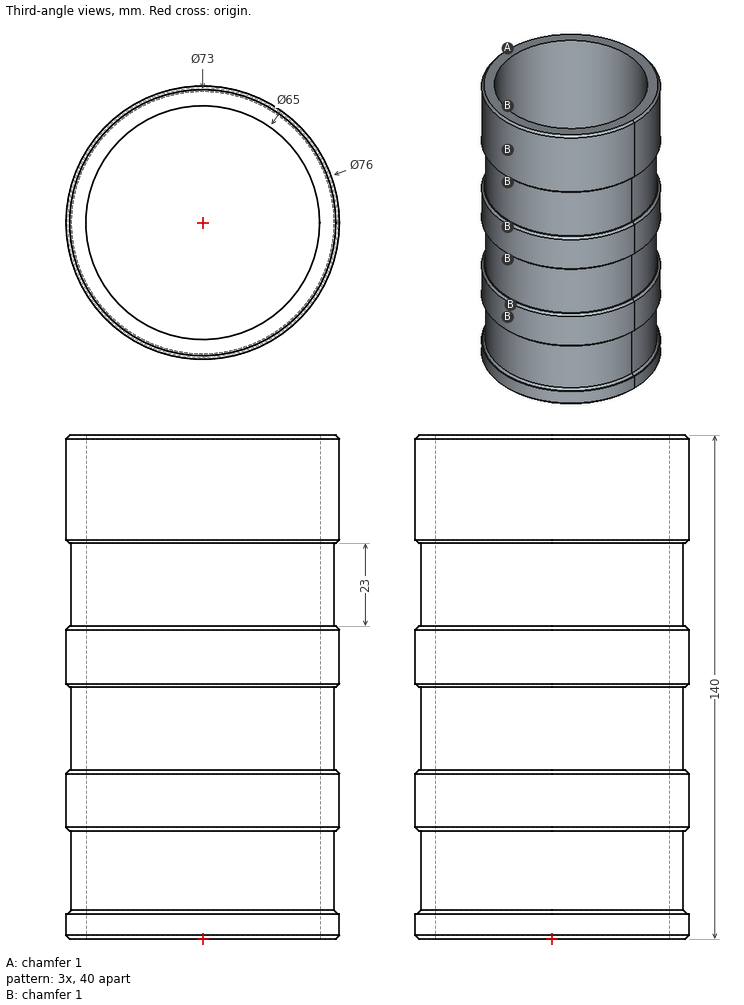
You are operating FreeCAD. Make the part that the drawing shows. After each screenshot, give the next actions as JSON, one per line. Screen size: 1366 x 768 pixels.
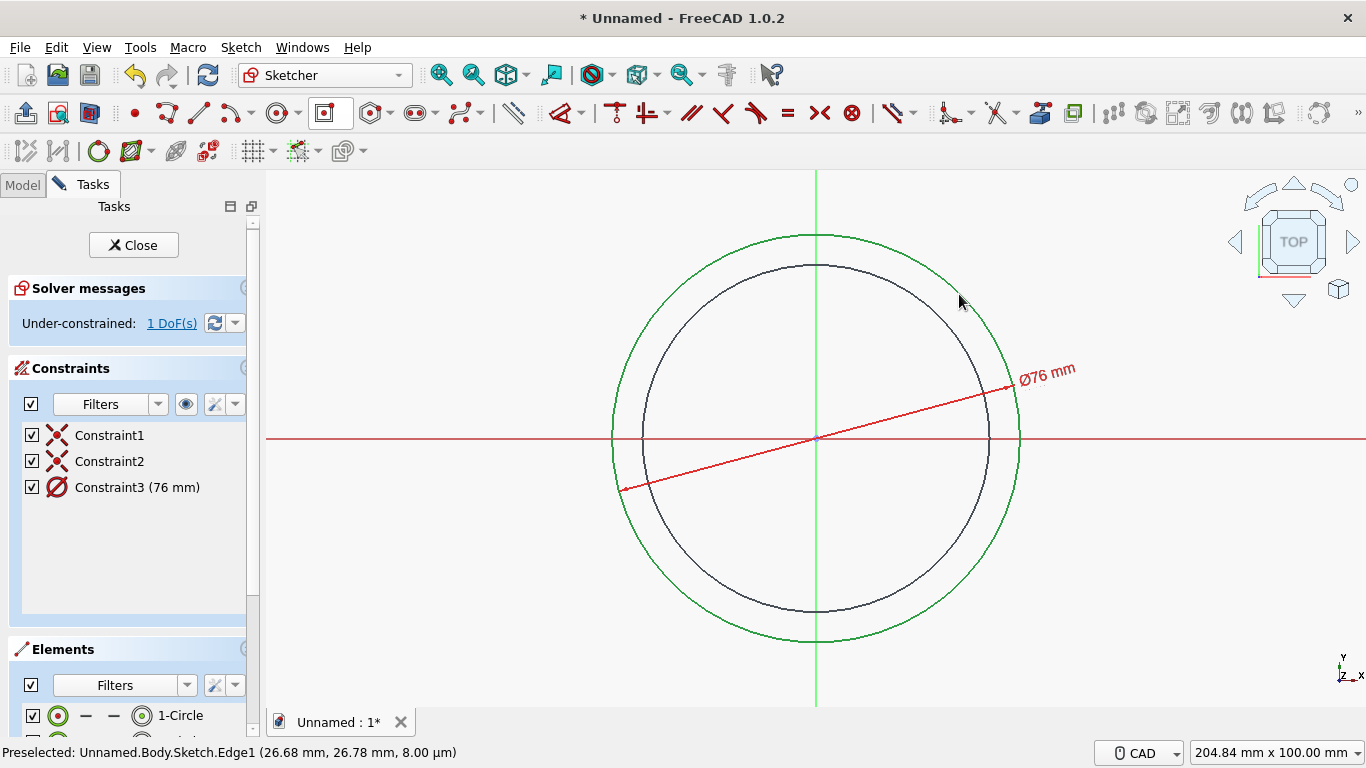
{"action": "left_click", "coordinate": [938, 315]}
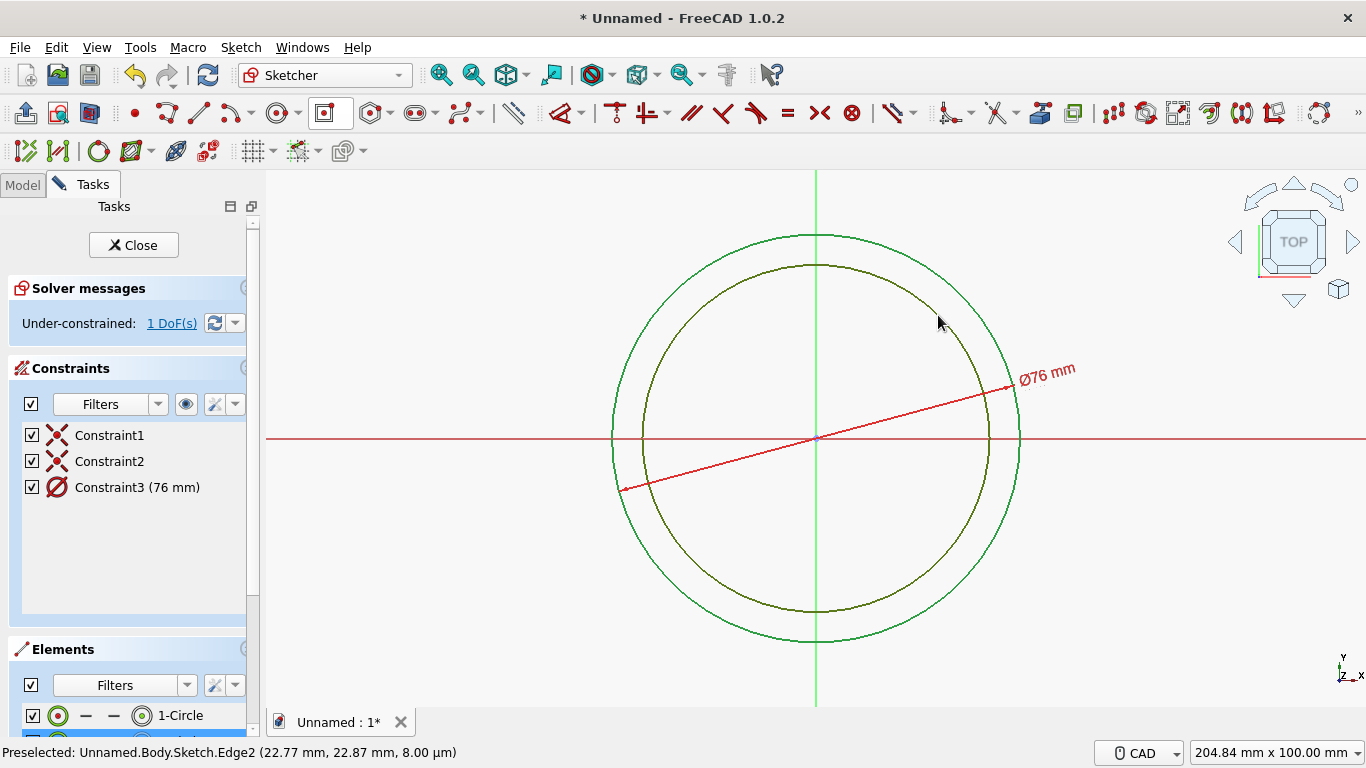
{"action": "key", "text": "k o"}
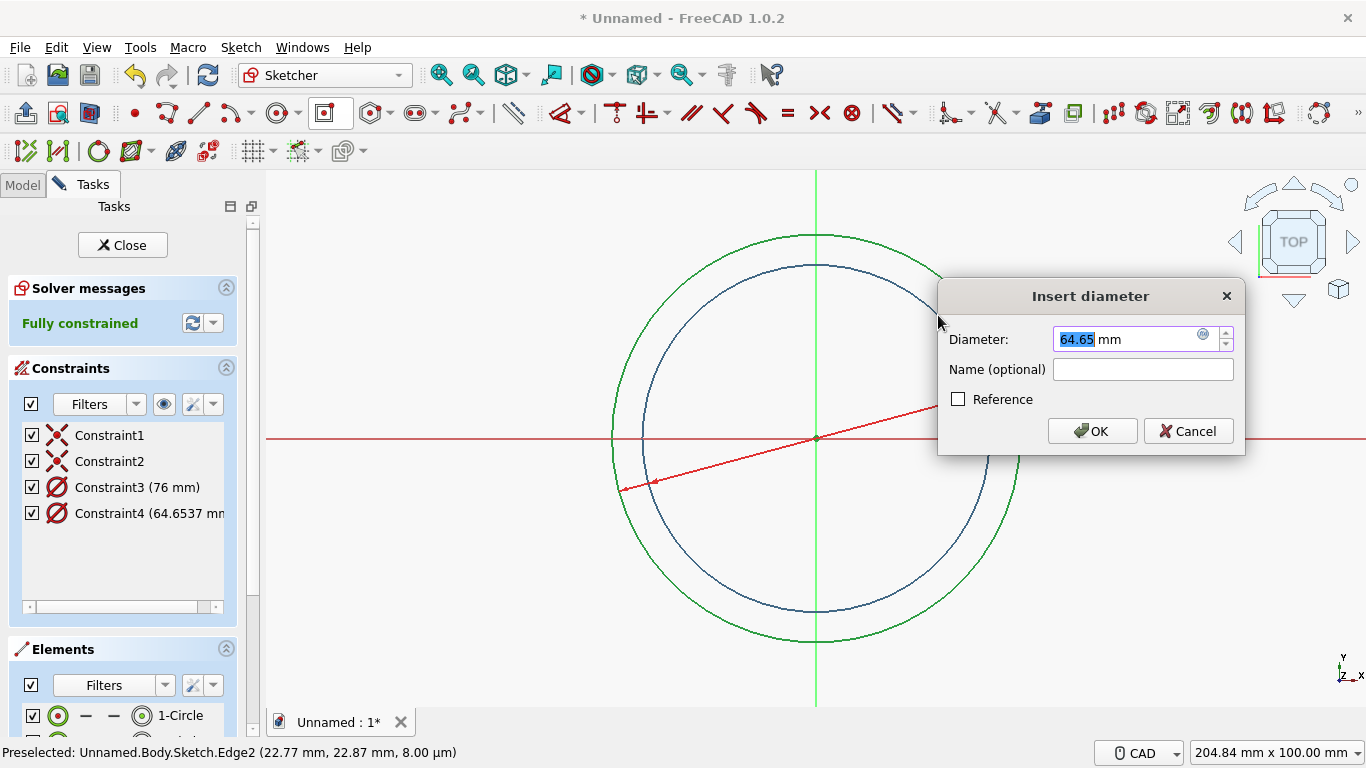
{"action": "type", "text": "65"}
{"action": "key", "text": "Return"}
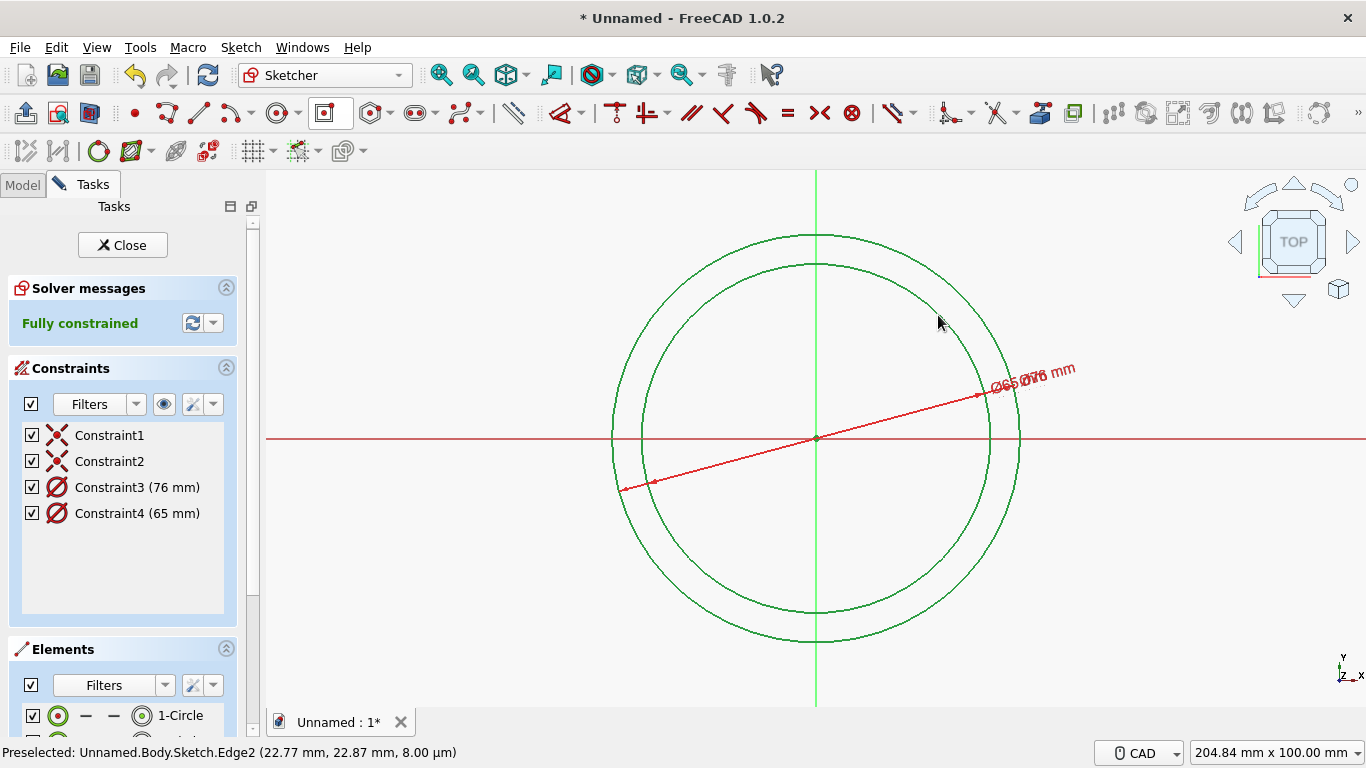
{"action": "left_click", "coordinate": [123, 245]}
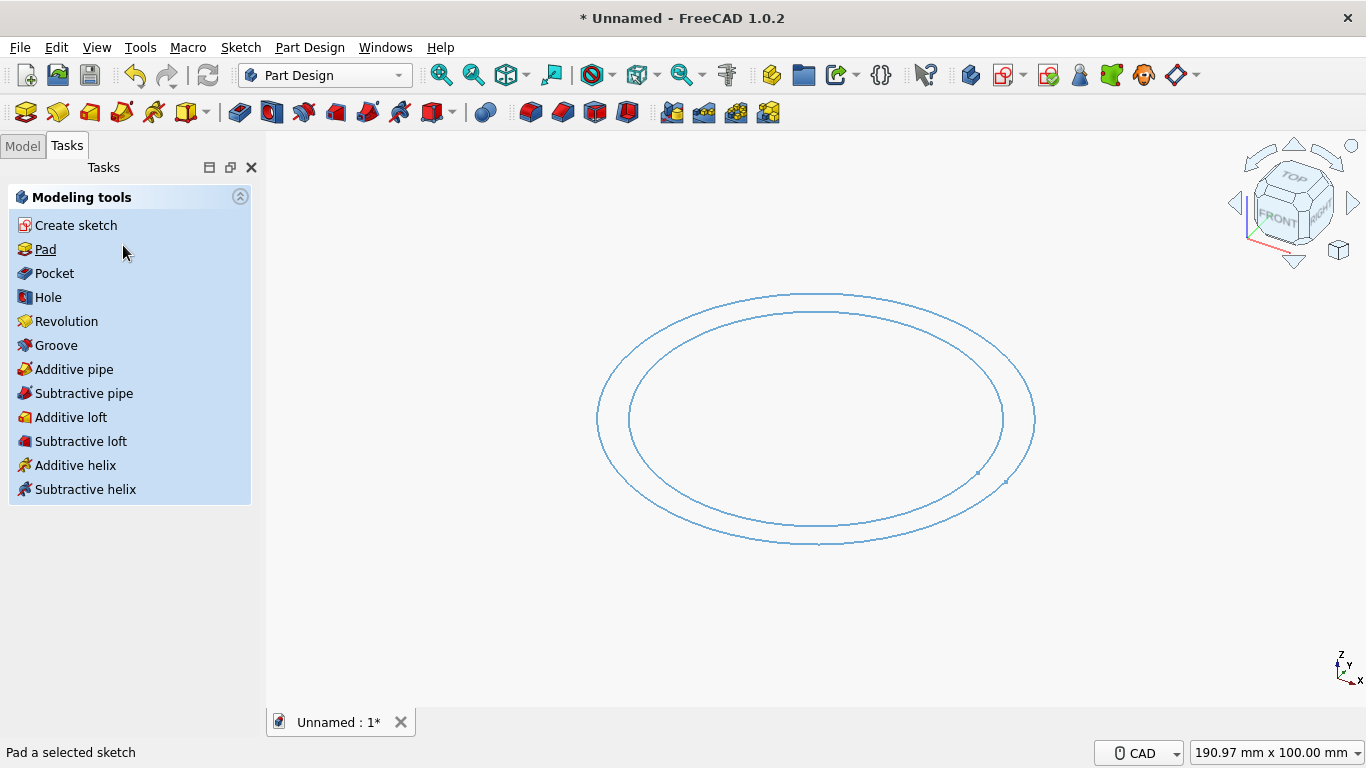
{"action": "left_click", "coordinate": [26, 112]}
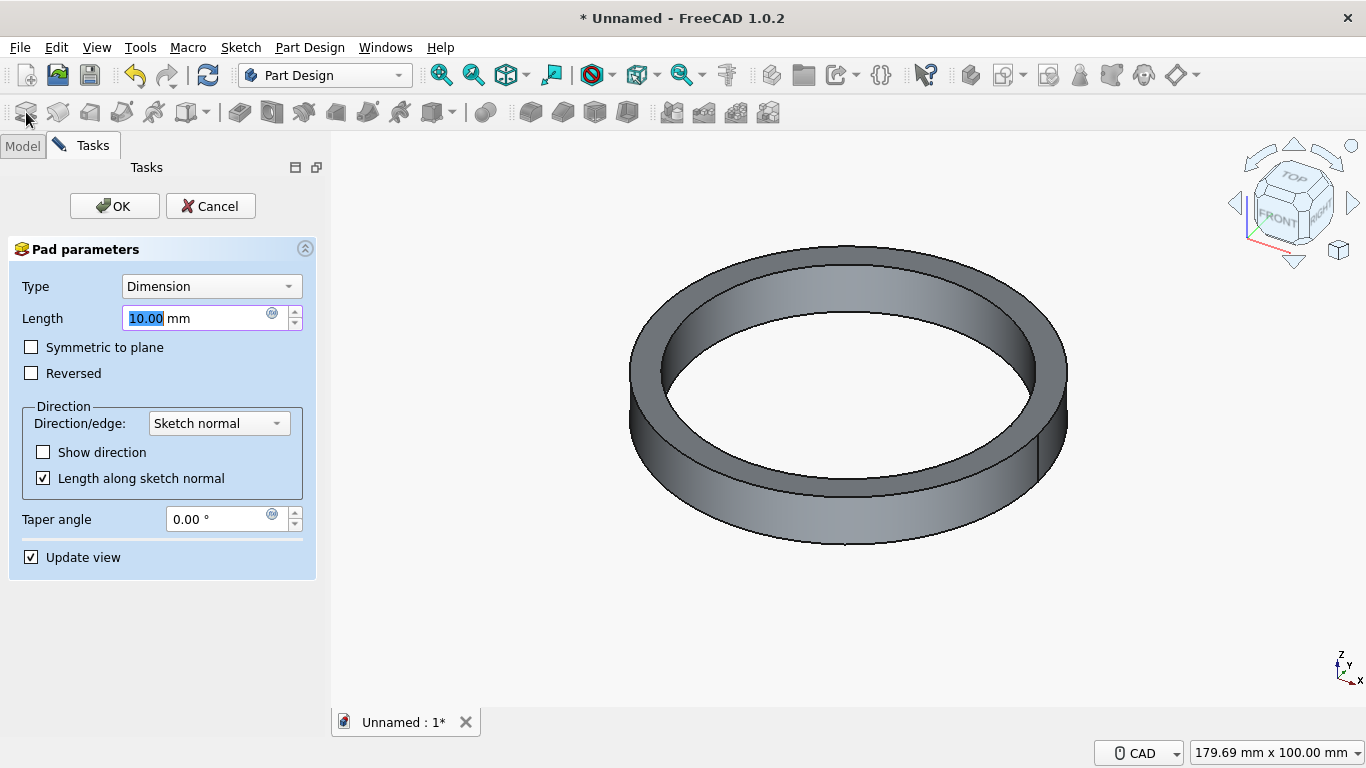
{"action": "type", "text": "140"}
{"action": "key", "text": "Tab"}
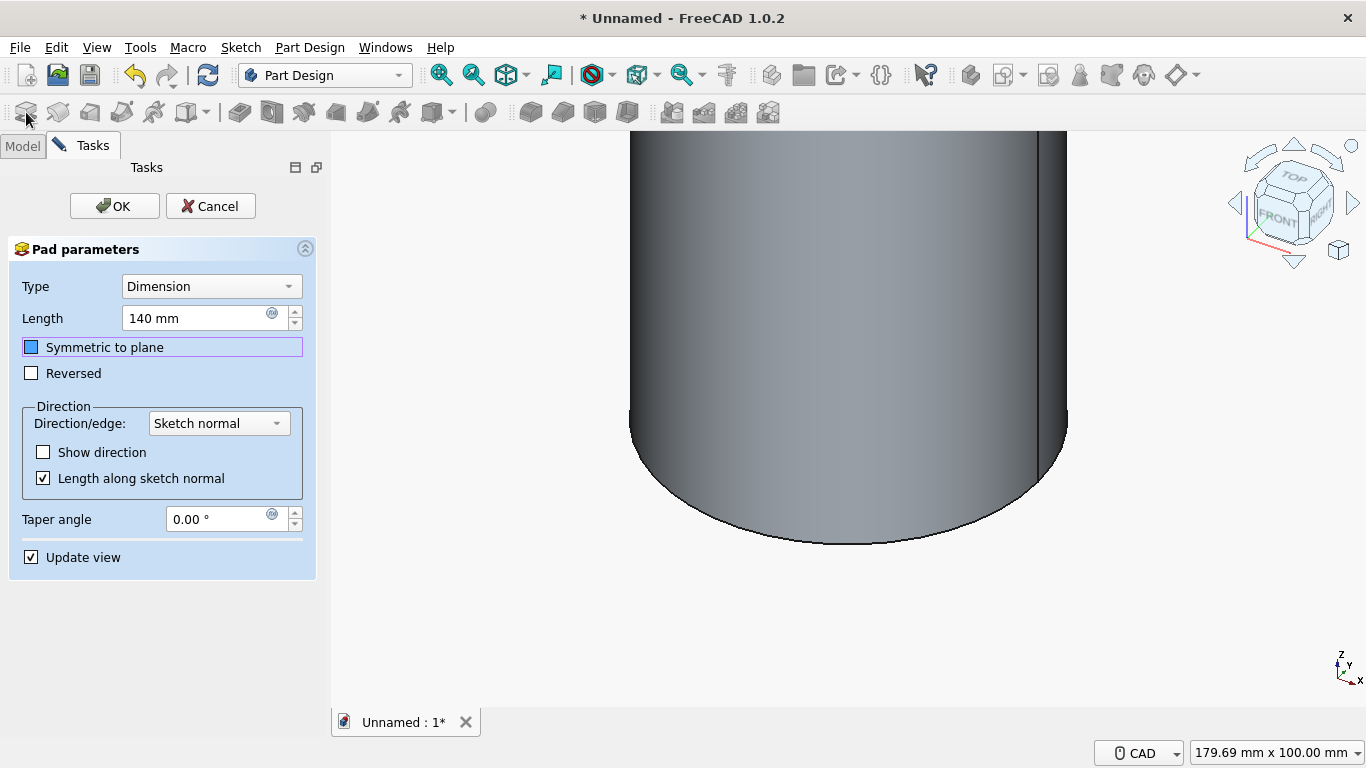
{"action": "left_click", "coordinate": [115, 206]}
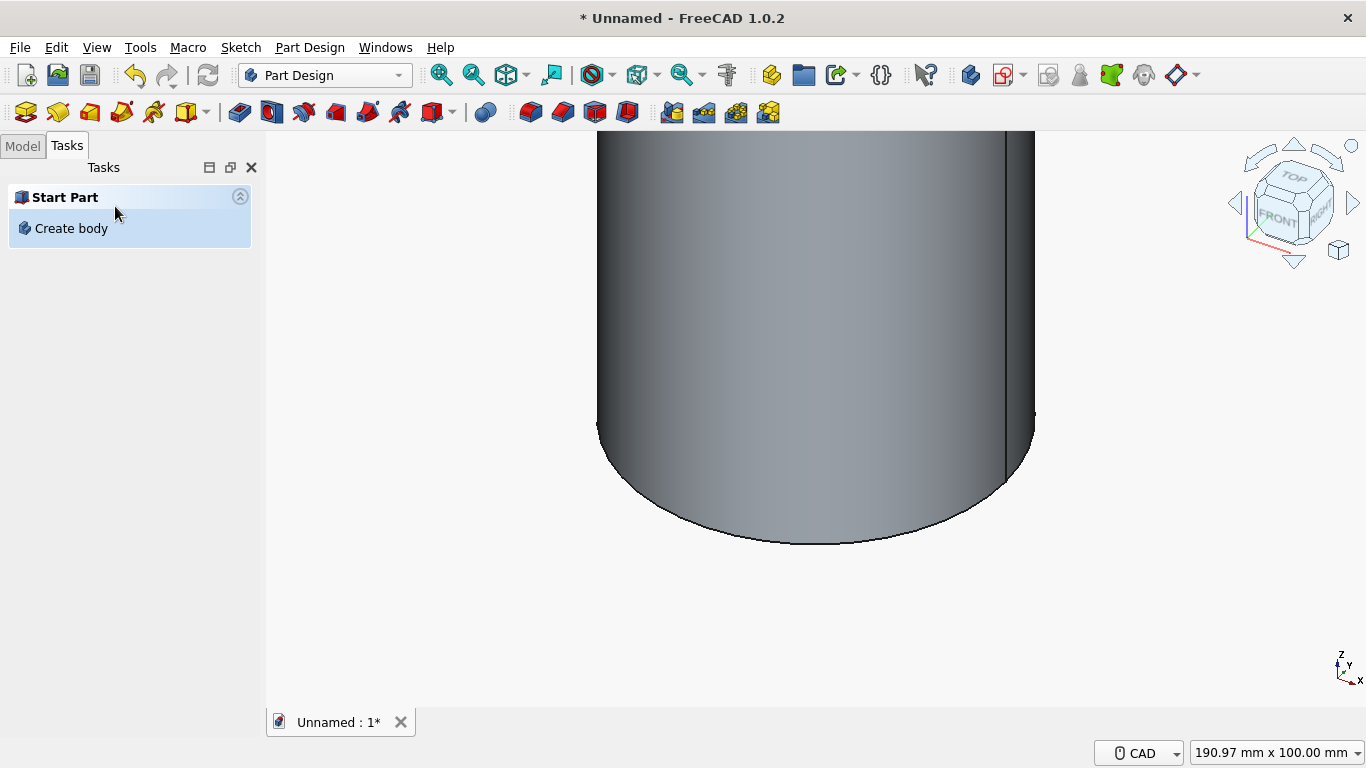
{"action": "key", "text": "v f"}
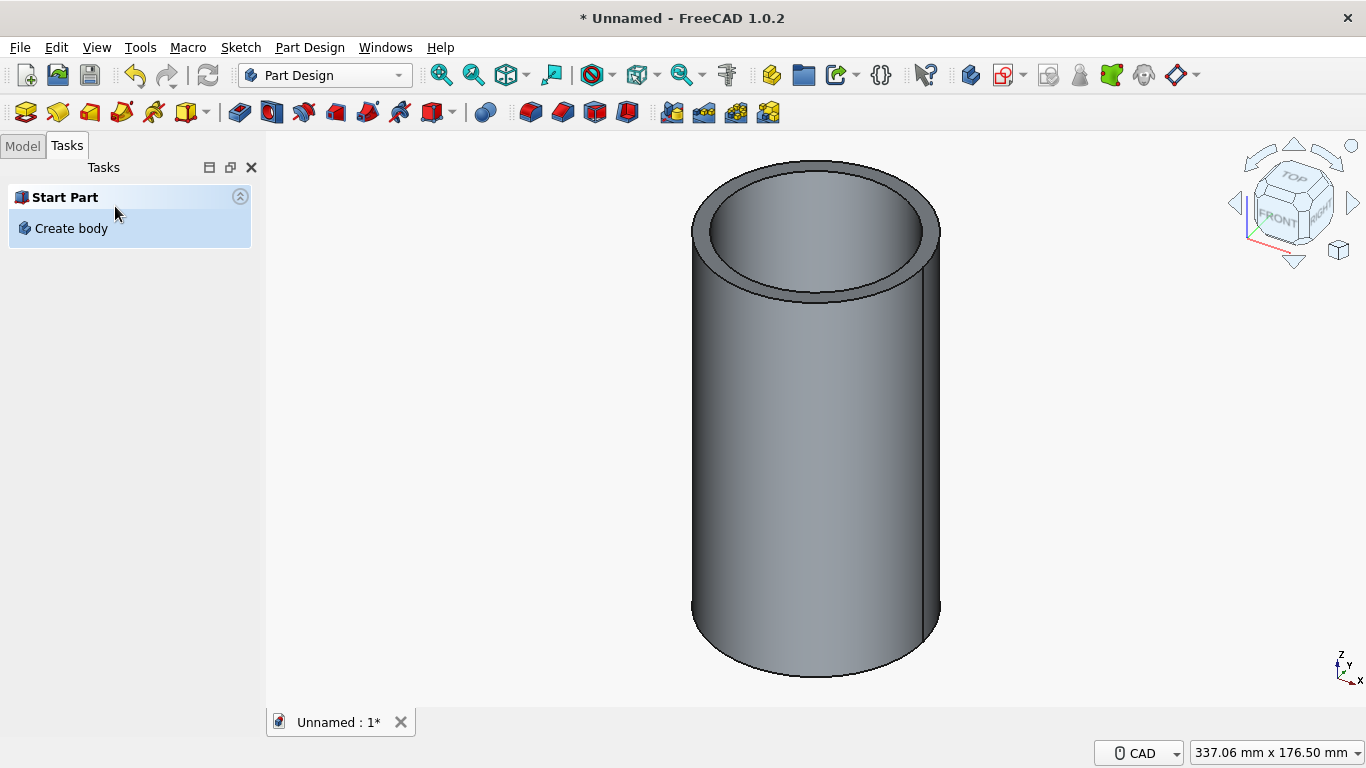
{"action": "left_click", "coordinate": [693, 238]}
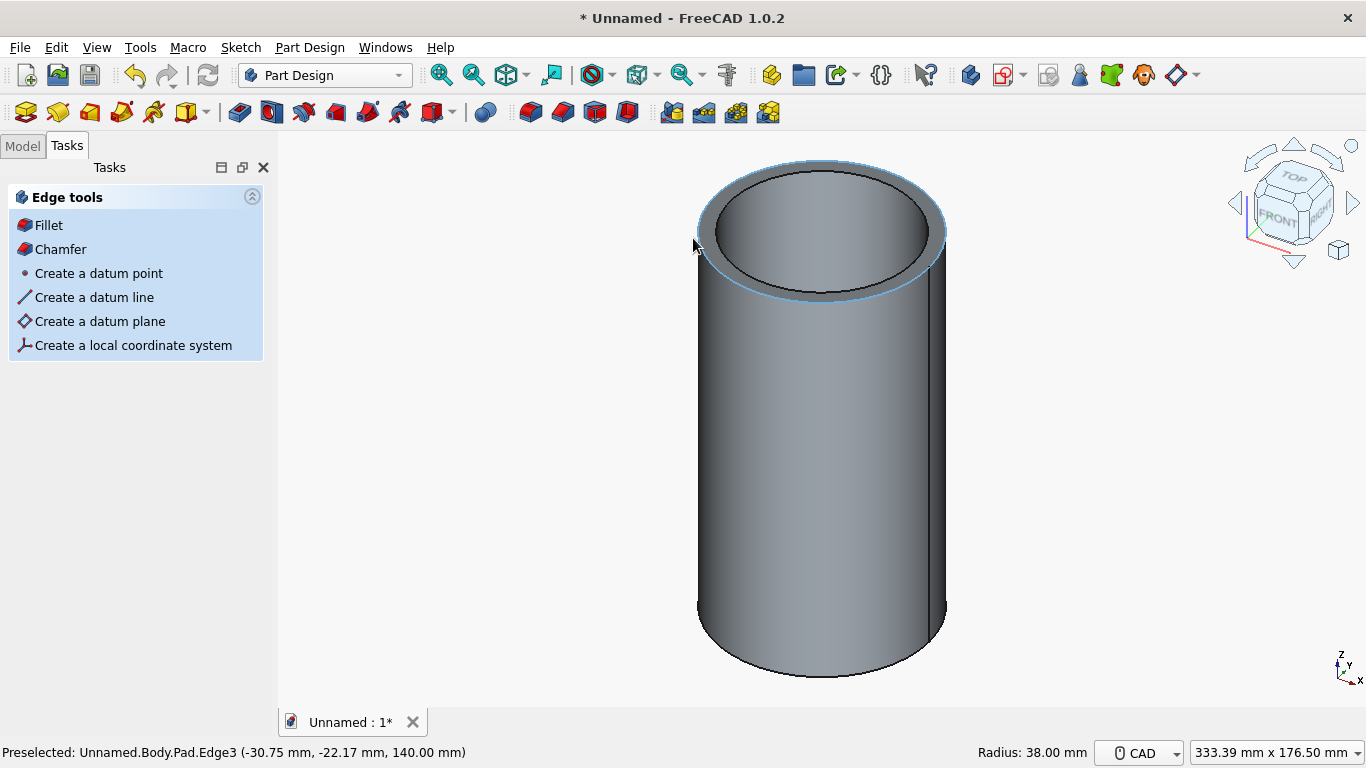
{"action": "left_click", "coordinate": [564, 112]}